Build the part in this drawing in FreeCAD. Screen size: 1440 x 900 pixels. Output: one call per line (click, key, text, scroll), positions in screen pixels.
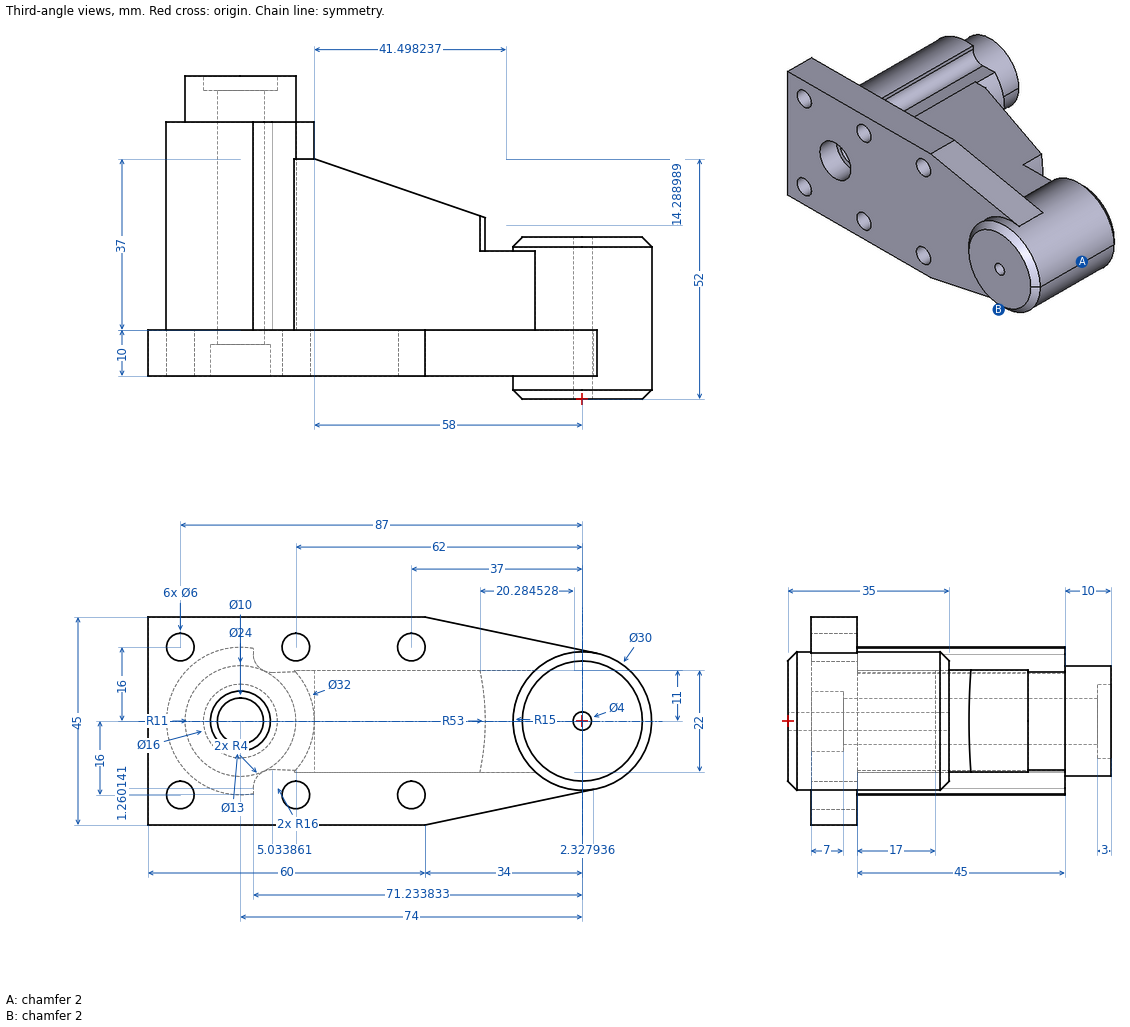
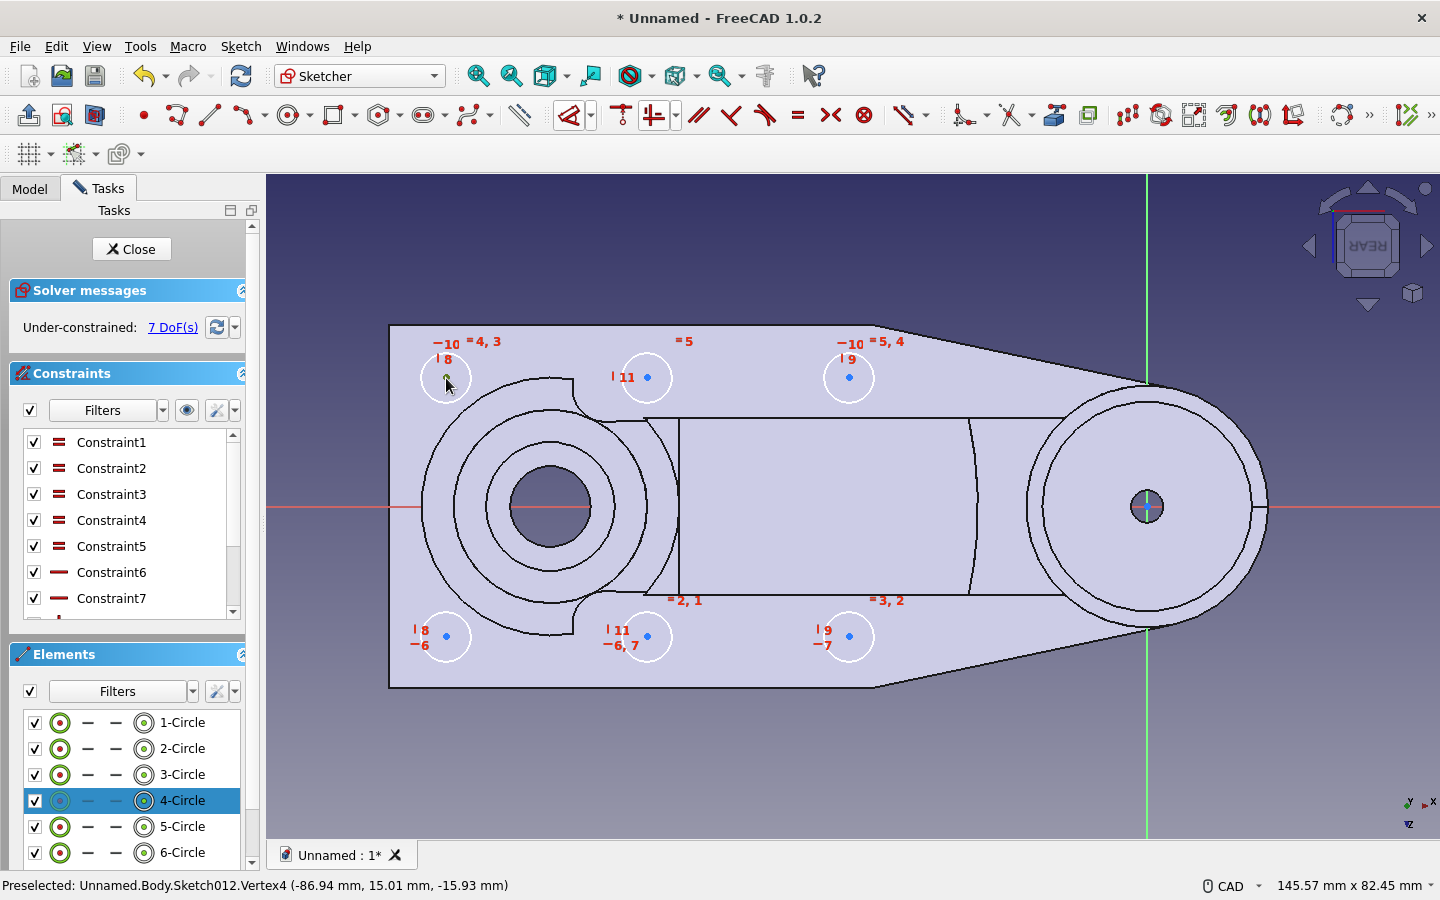
click(647, 378)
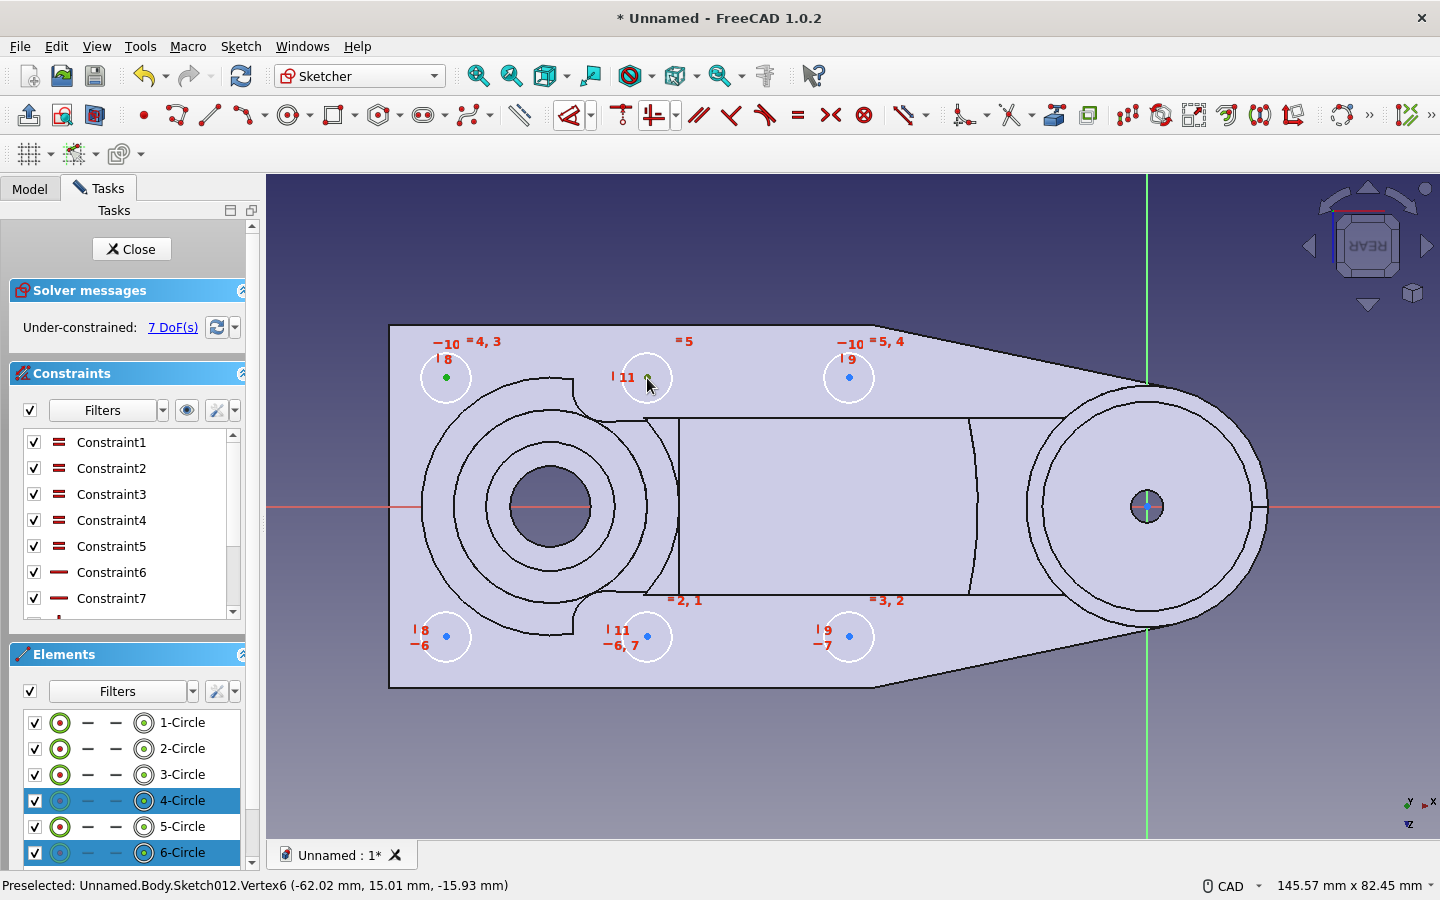
key(h)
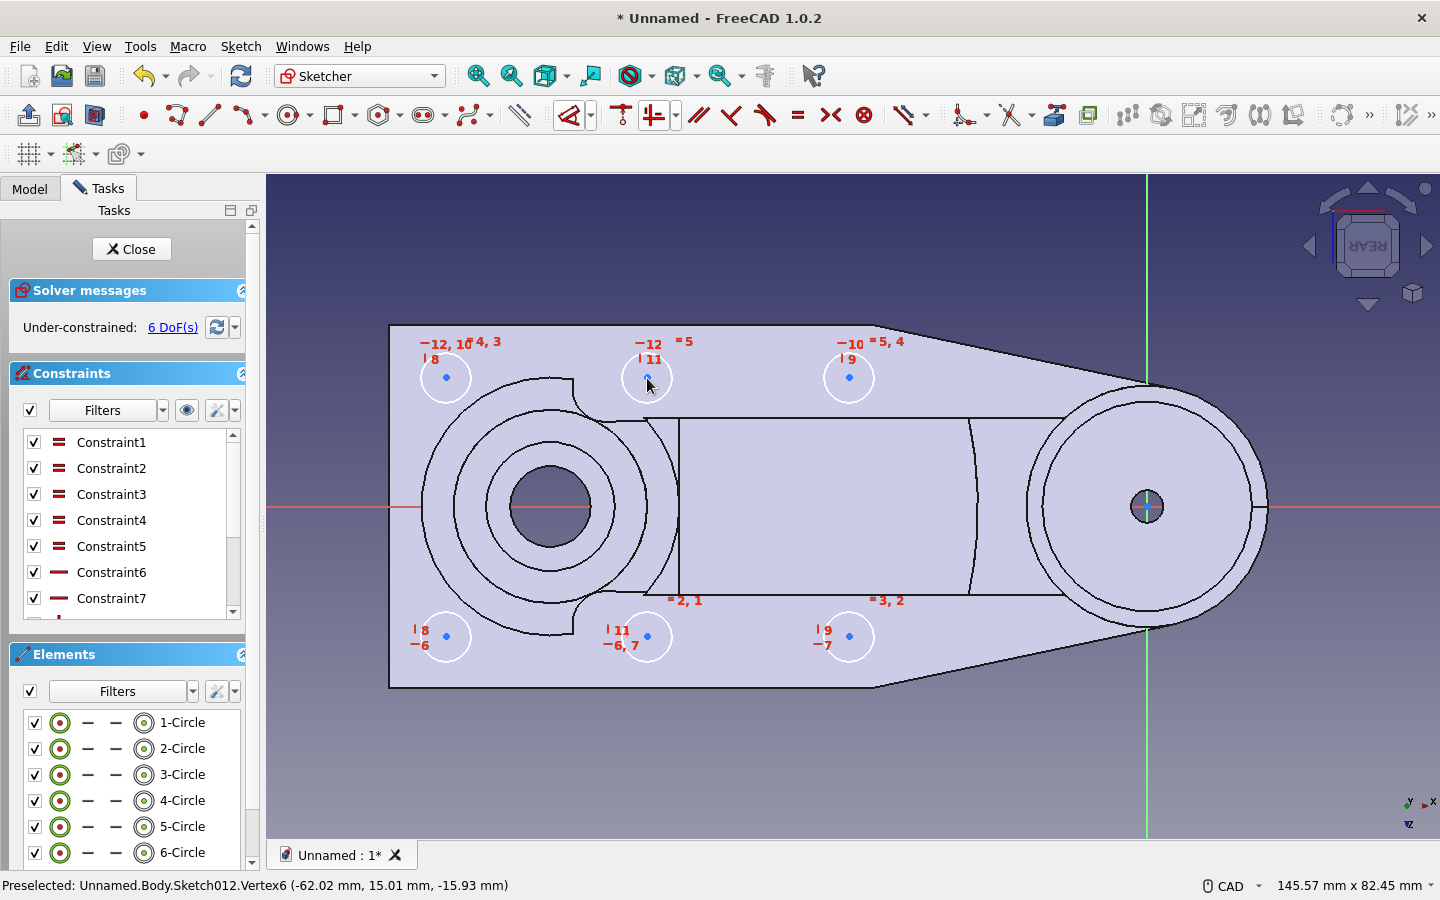
click(463, 619)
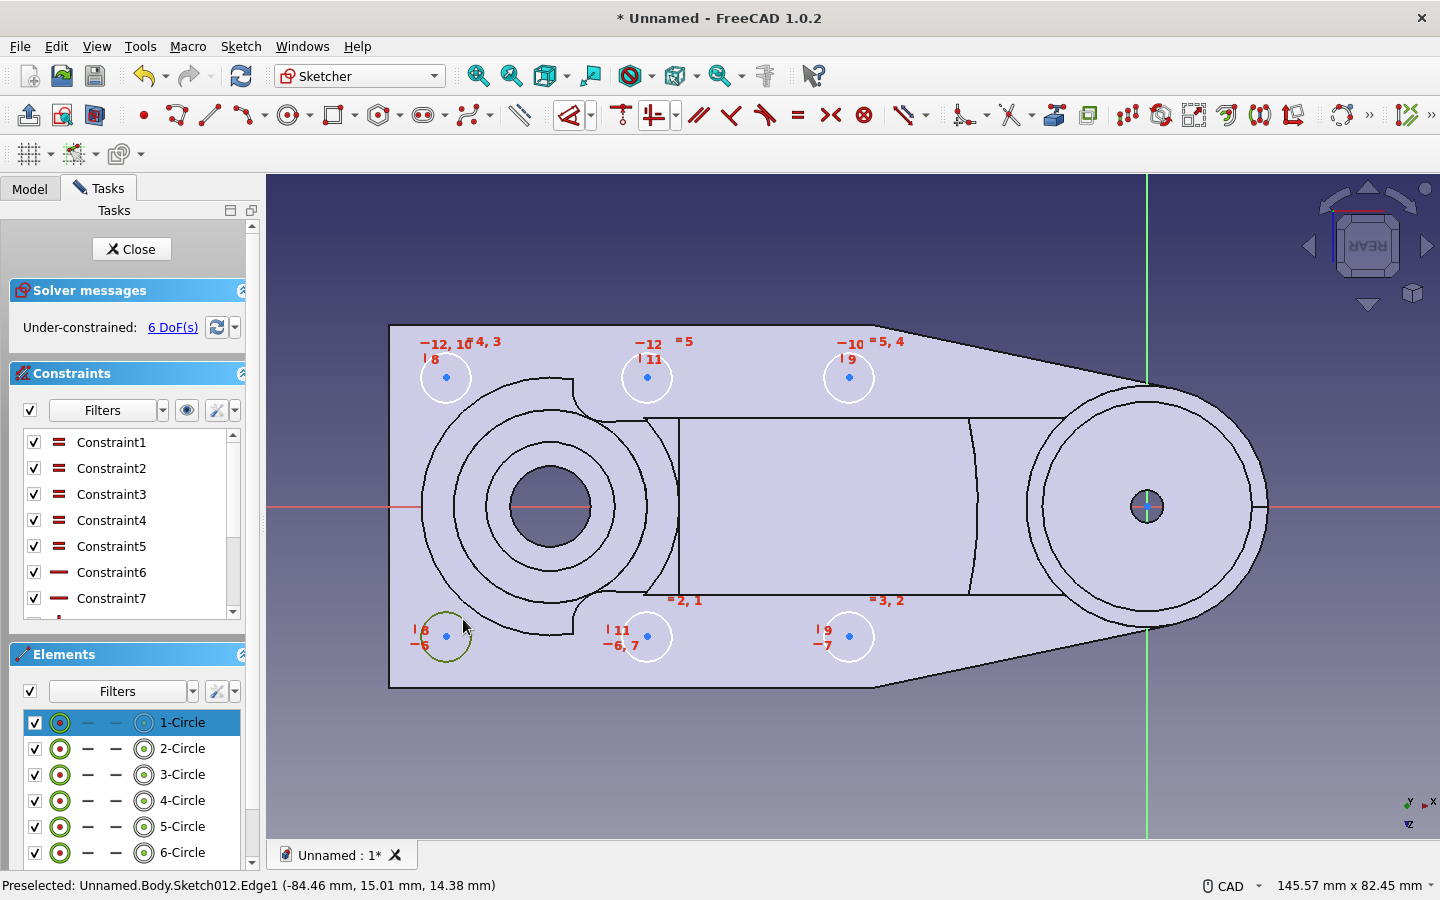
click(590, 116)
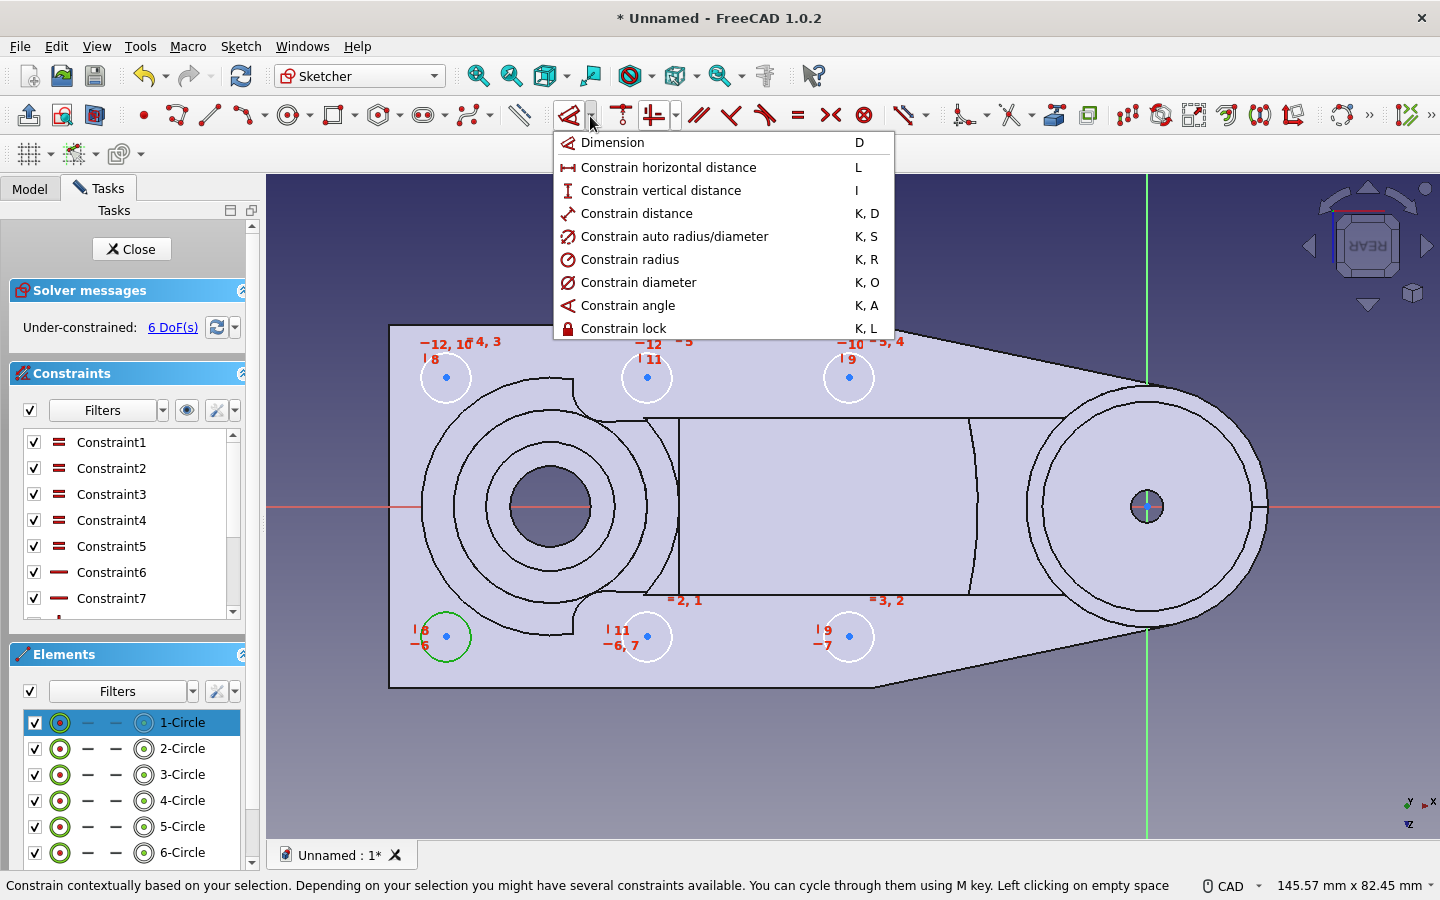
click(724, 282)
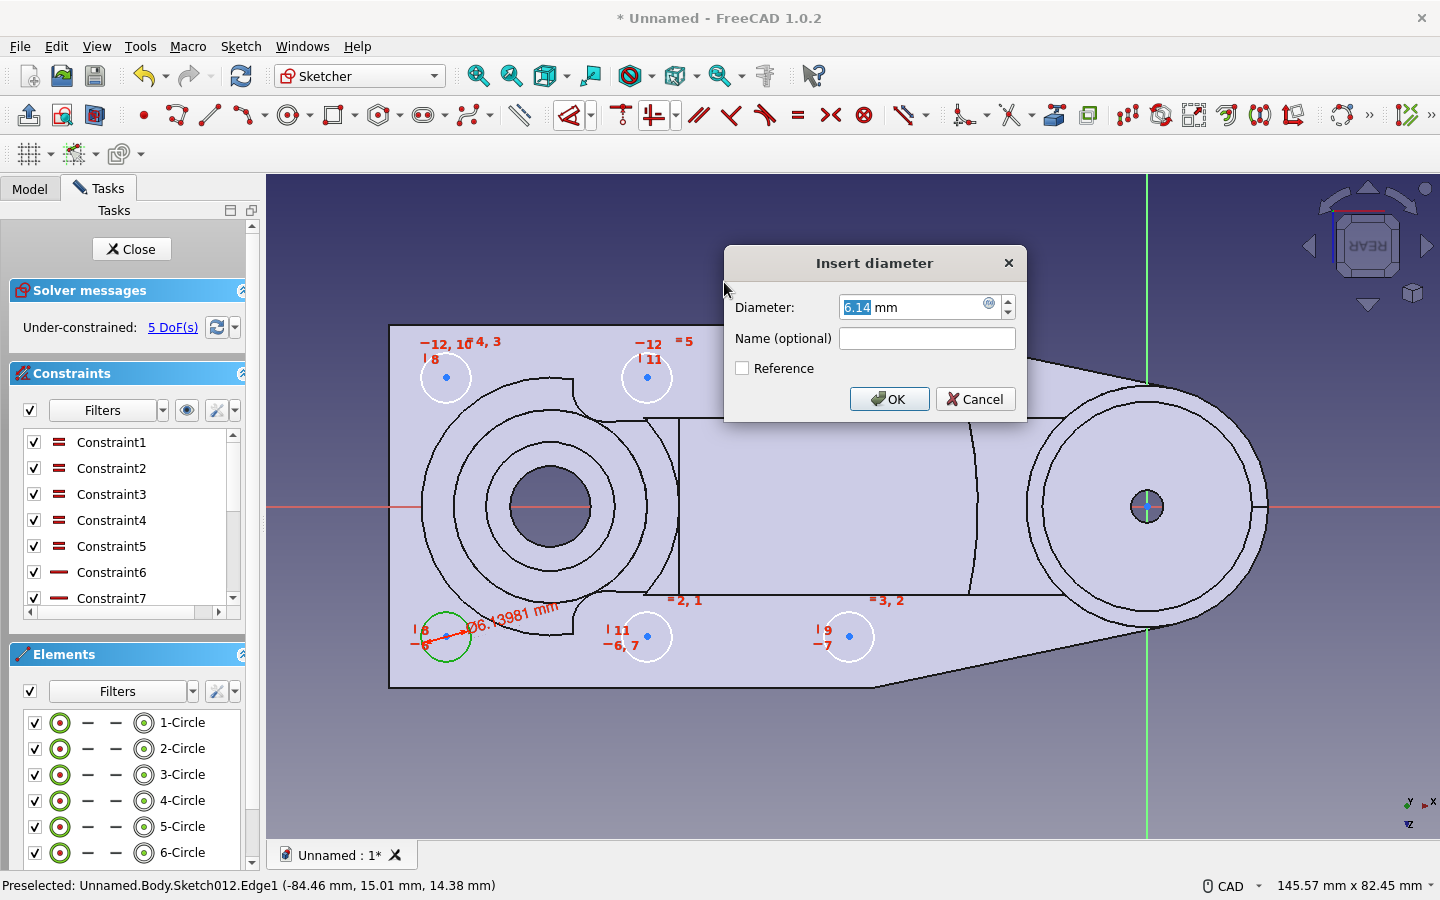
text(6)
key(Return)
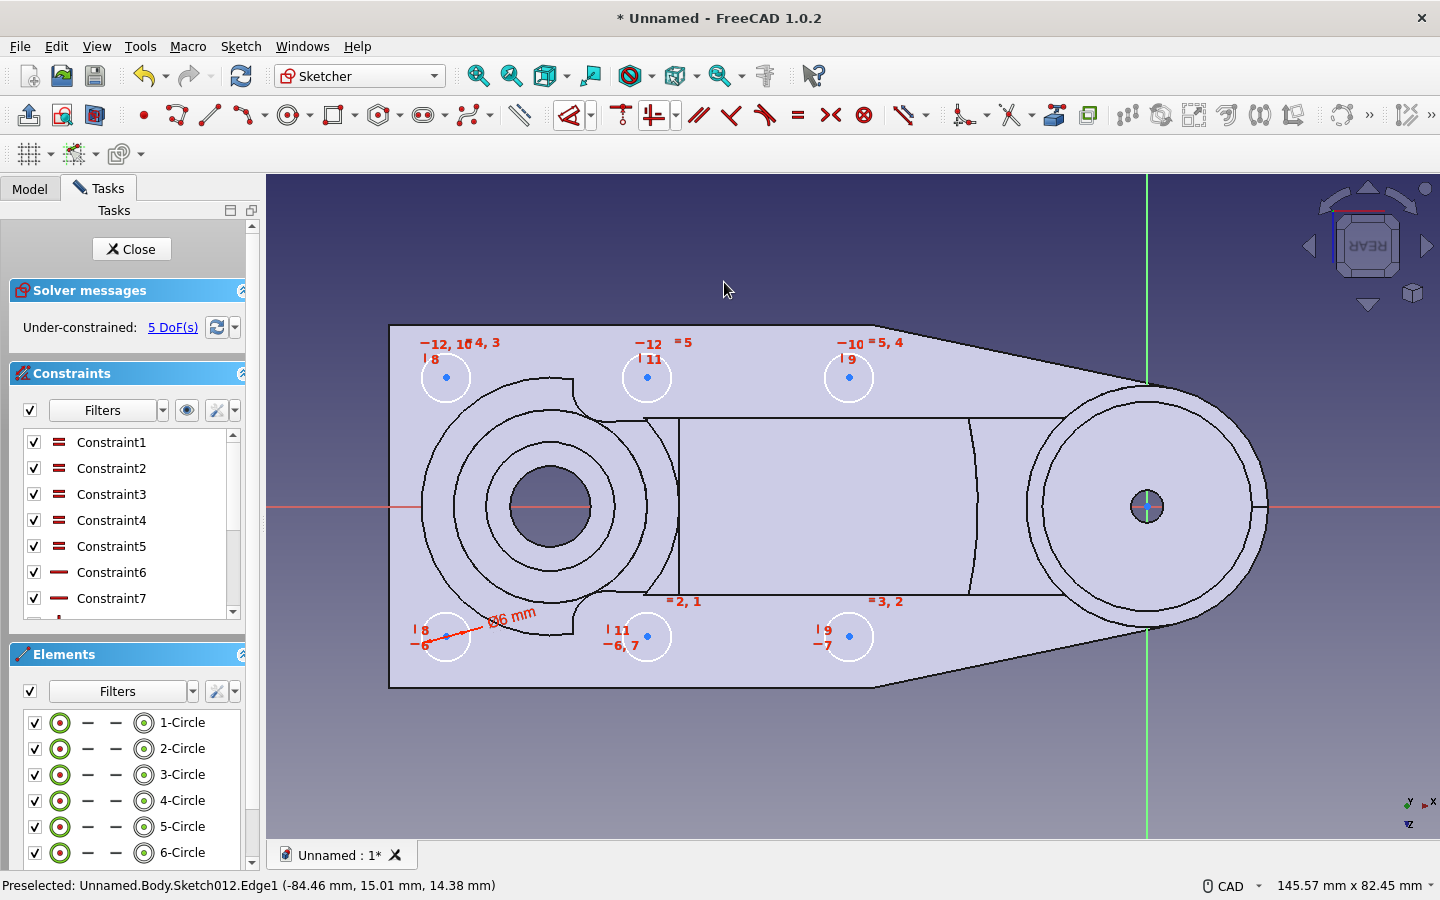
click(446, 637)